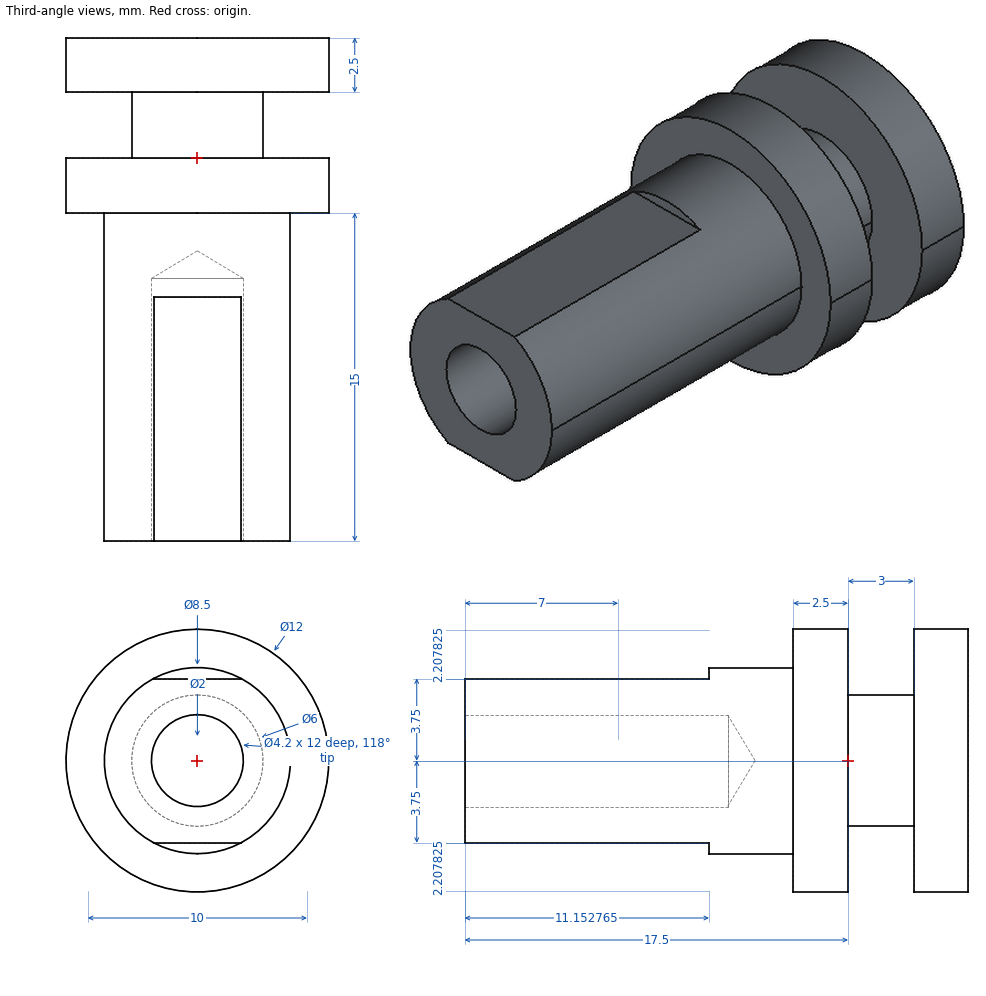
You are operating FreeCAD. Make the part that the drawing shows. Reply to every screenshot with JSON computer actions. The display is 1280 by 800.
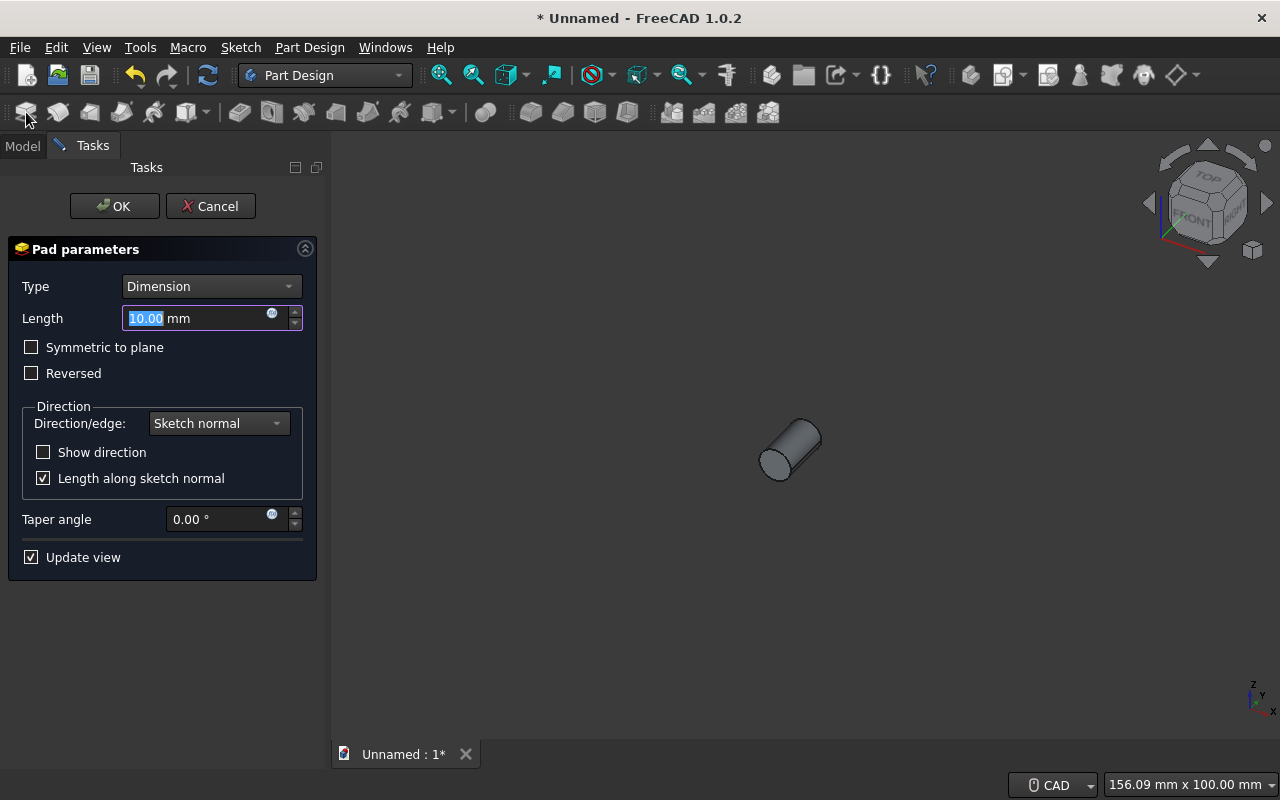
{"action": "type", "text": "3"}
{"action": "key", "text": "Tab"}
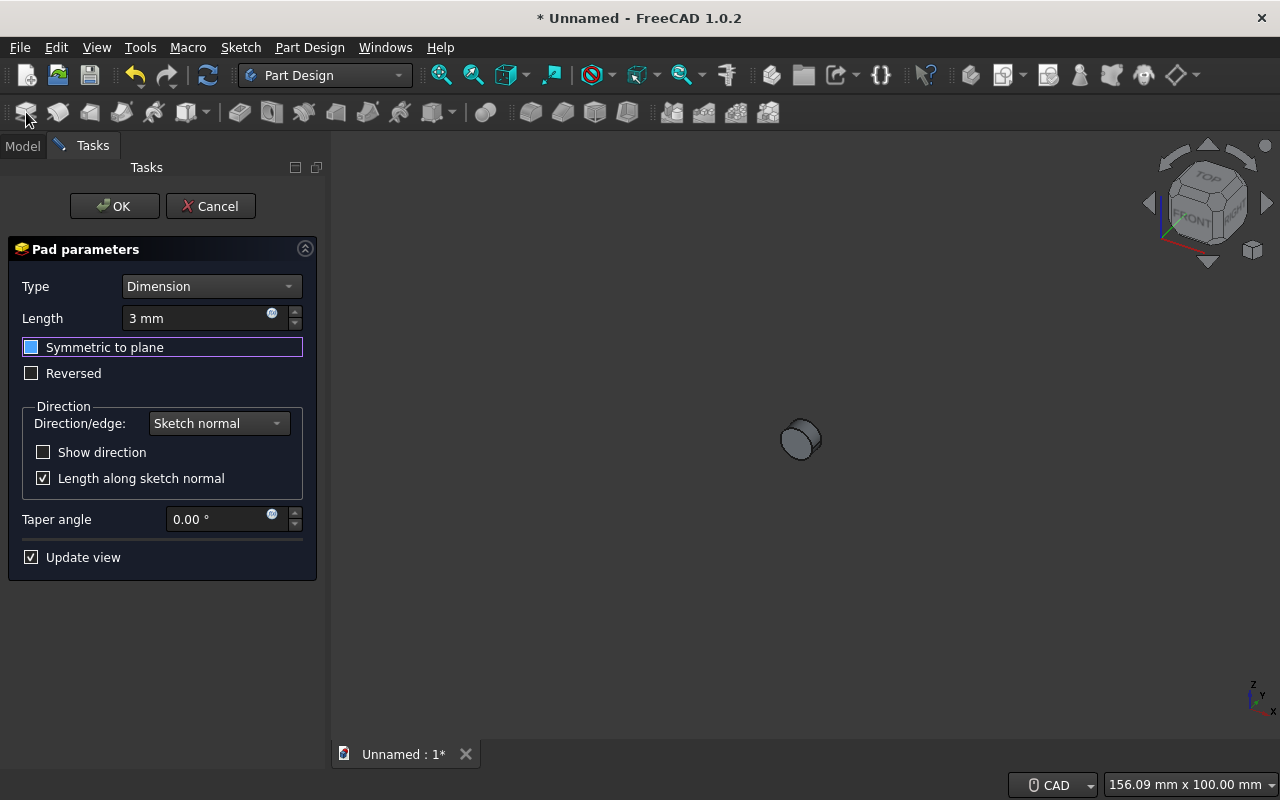
{"action": "left_click", "coordinate": [30, 373]}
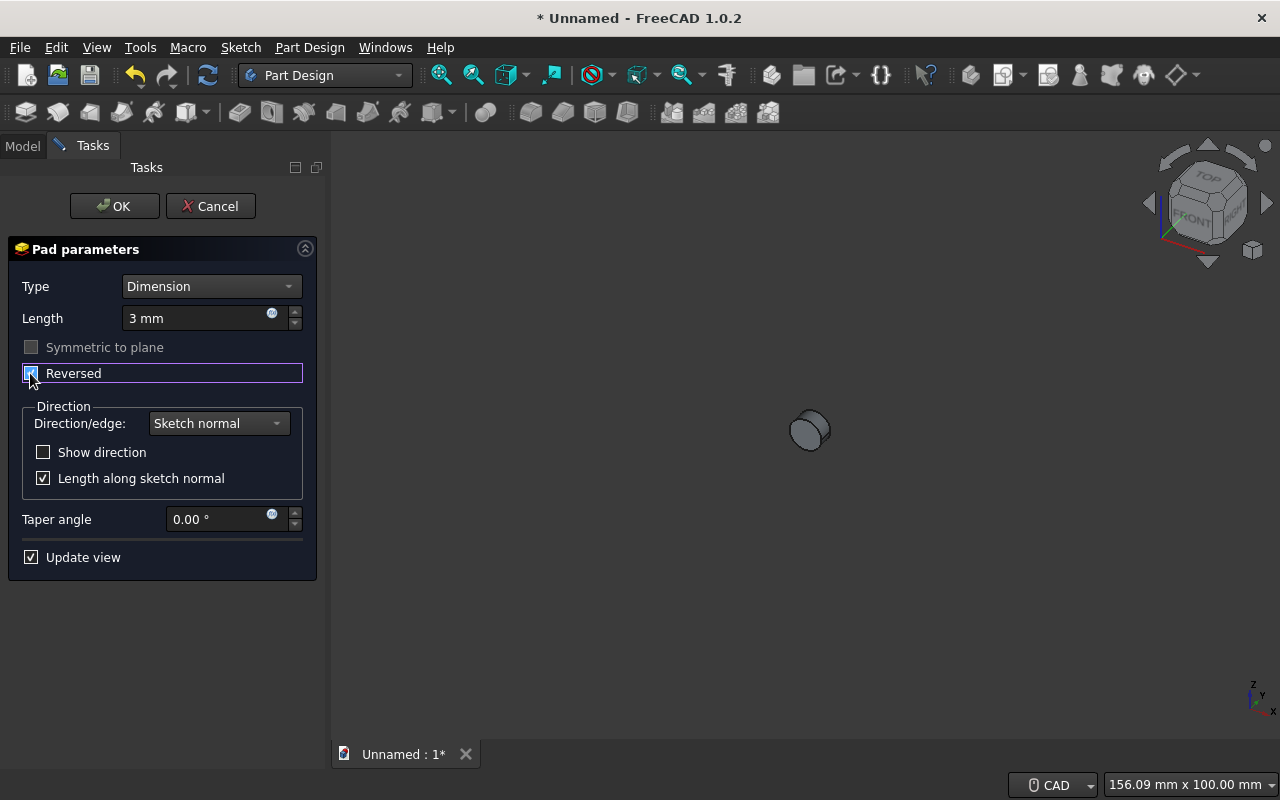
{"action": "left_click", "coordinate": [115, 206]}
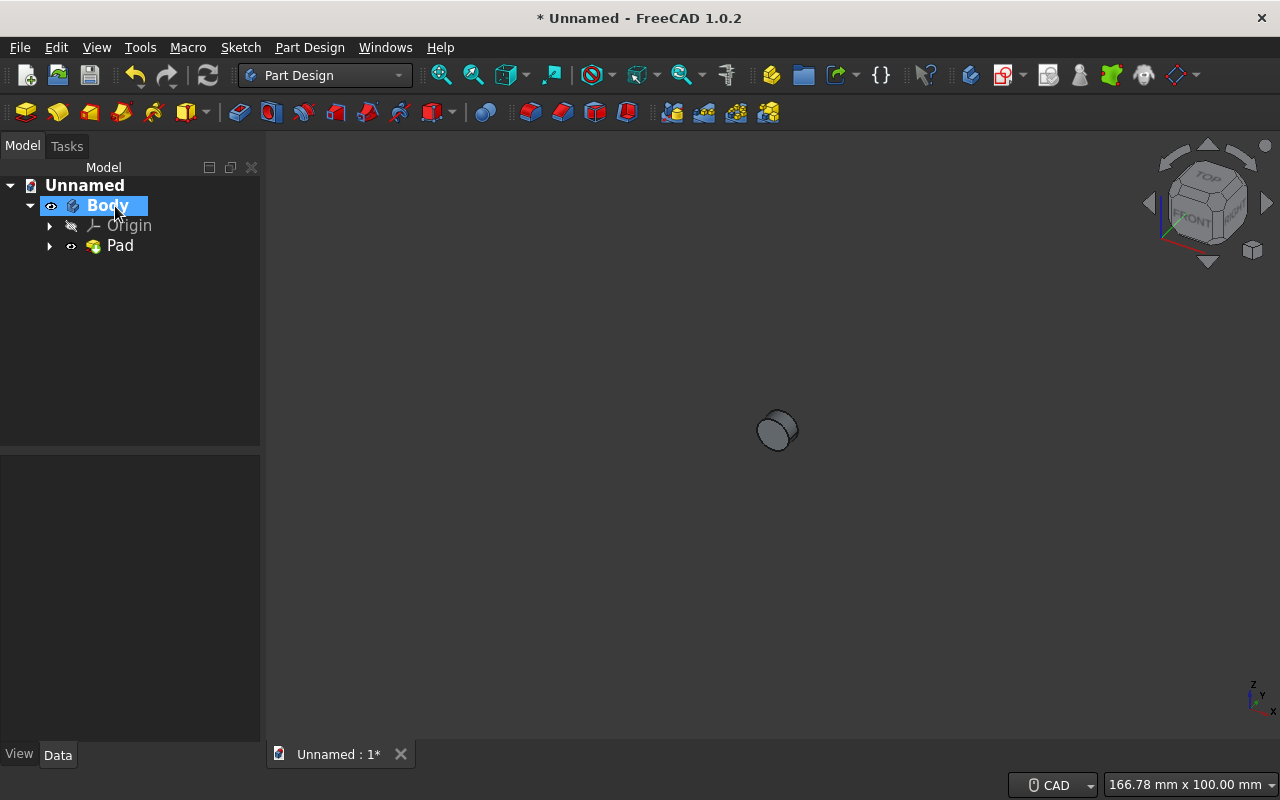
{"action": "key", "text": "v f"}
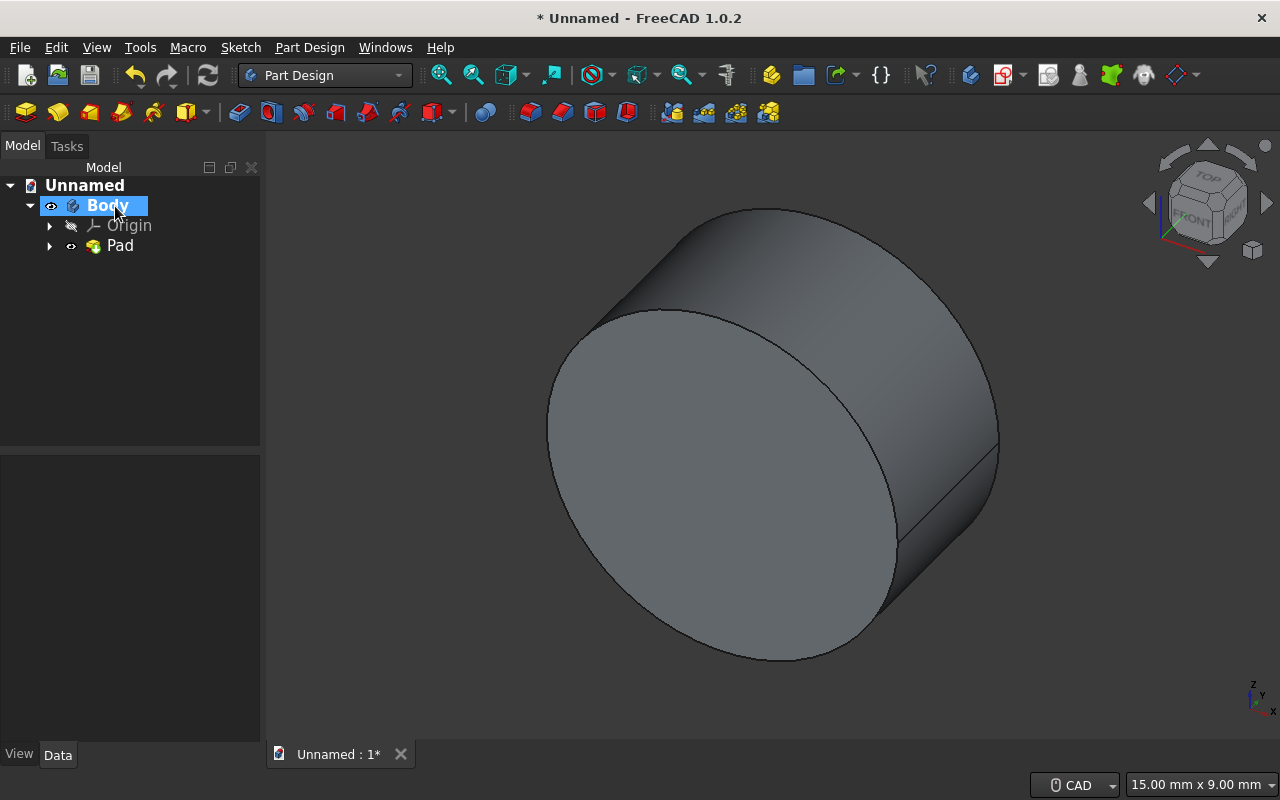
{"action": "key", "text": "4"}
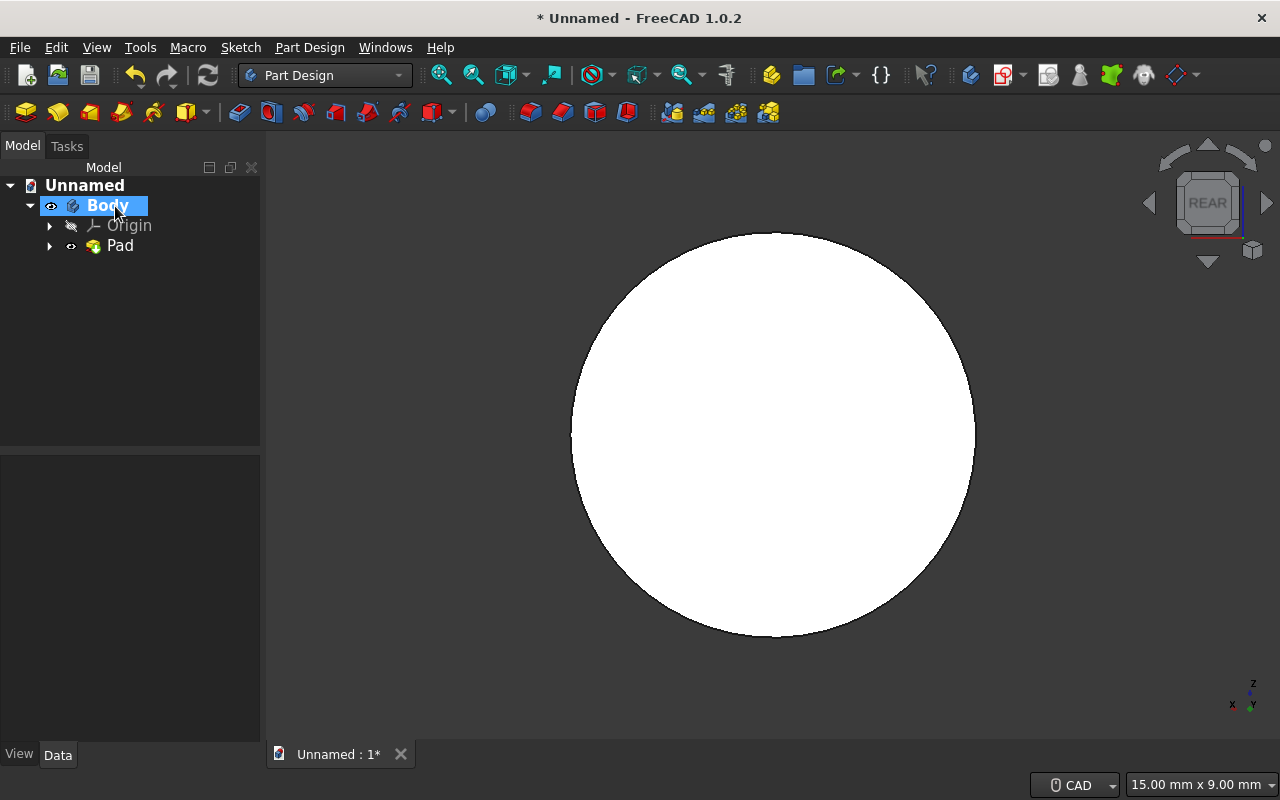
{"action": "left_click", "coordinate": [773, 434]}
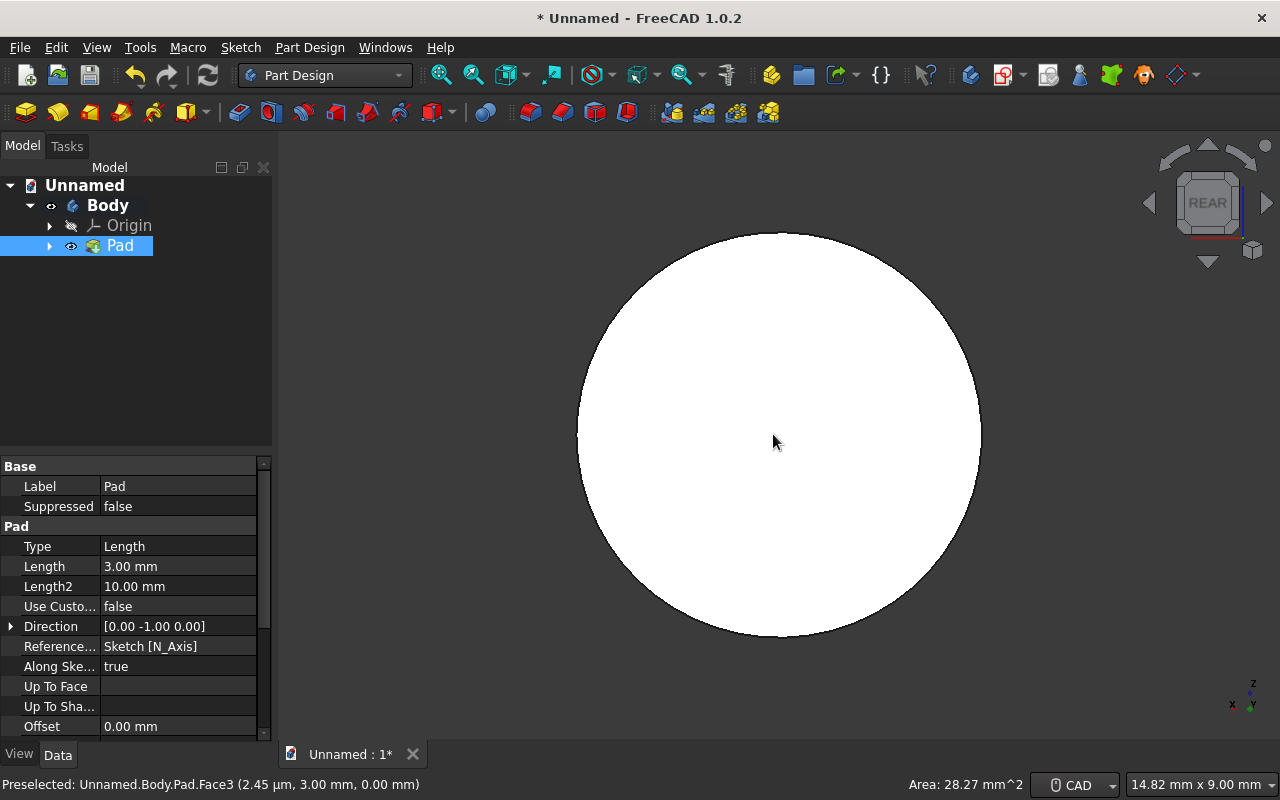
{"action": "left_click", "coordinate": [1004, 76]}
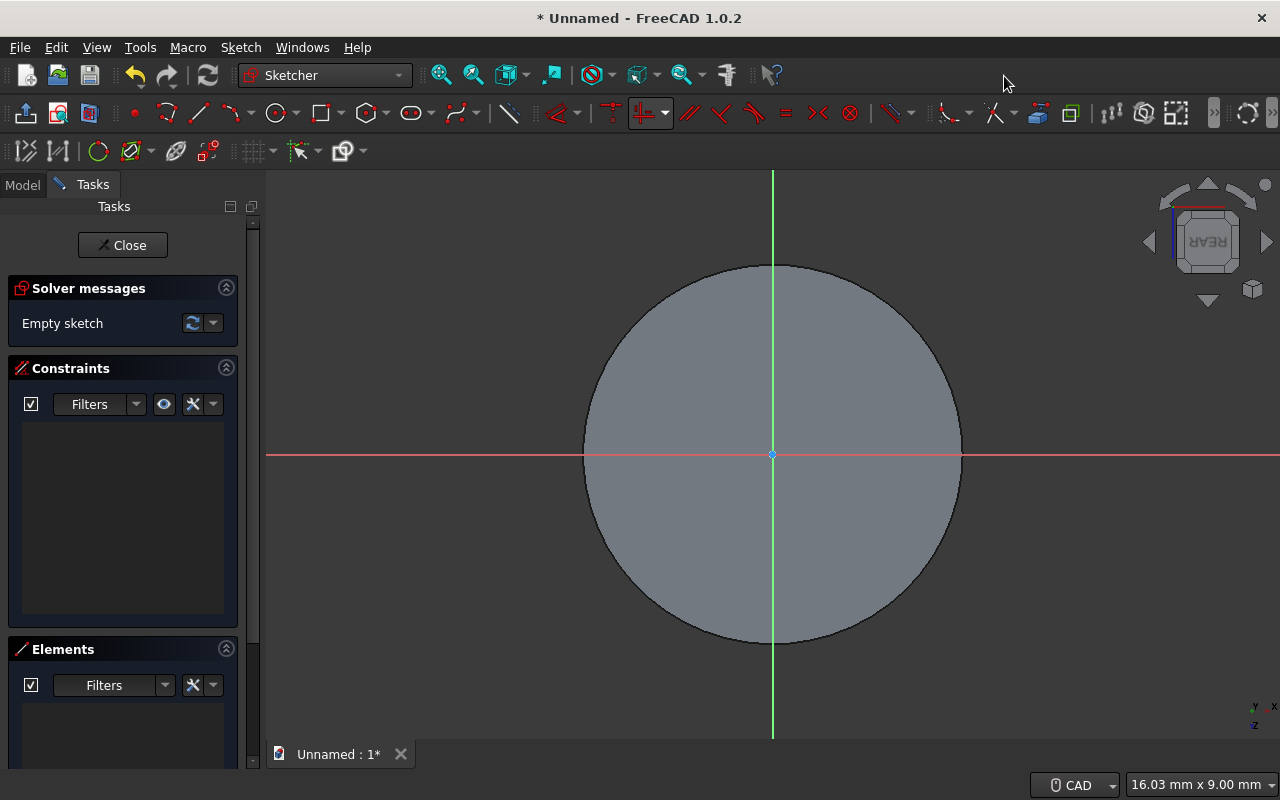
{"action": "scroll", "coordinate": [649, 454], "scroll_direction": "down", "scroll_amount": 4}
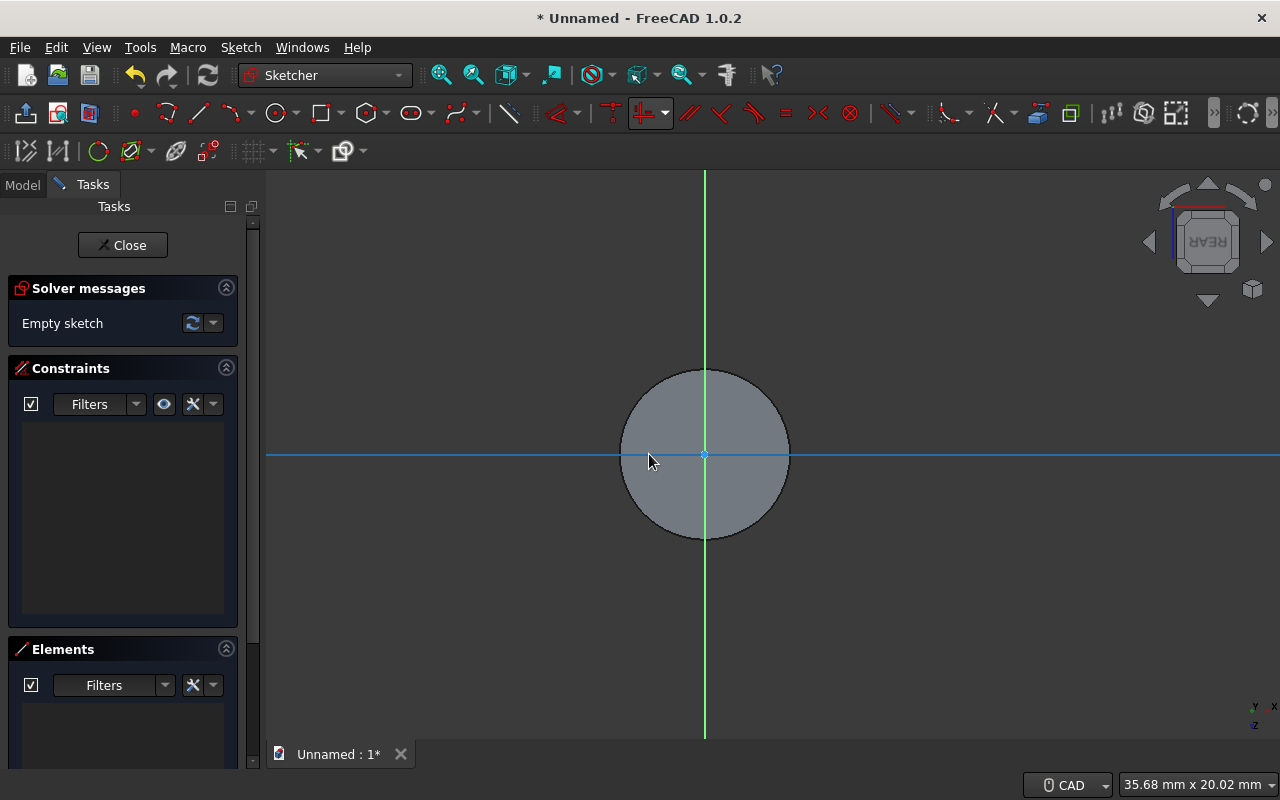
{"action": "key", "text": "g c"}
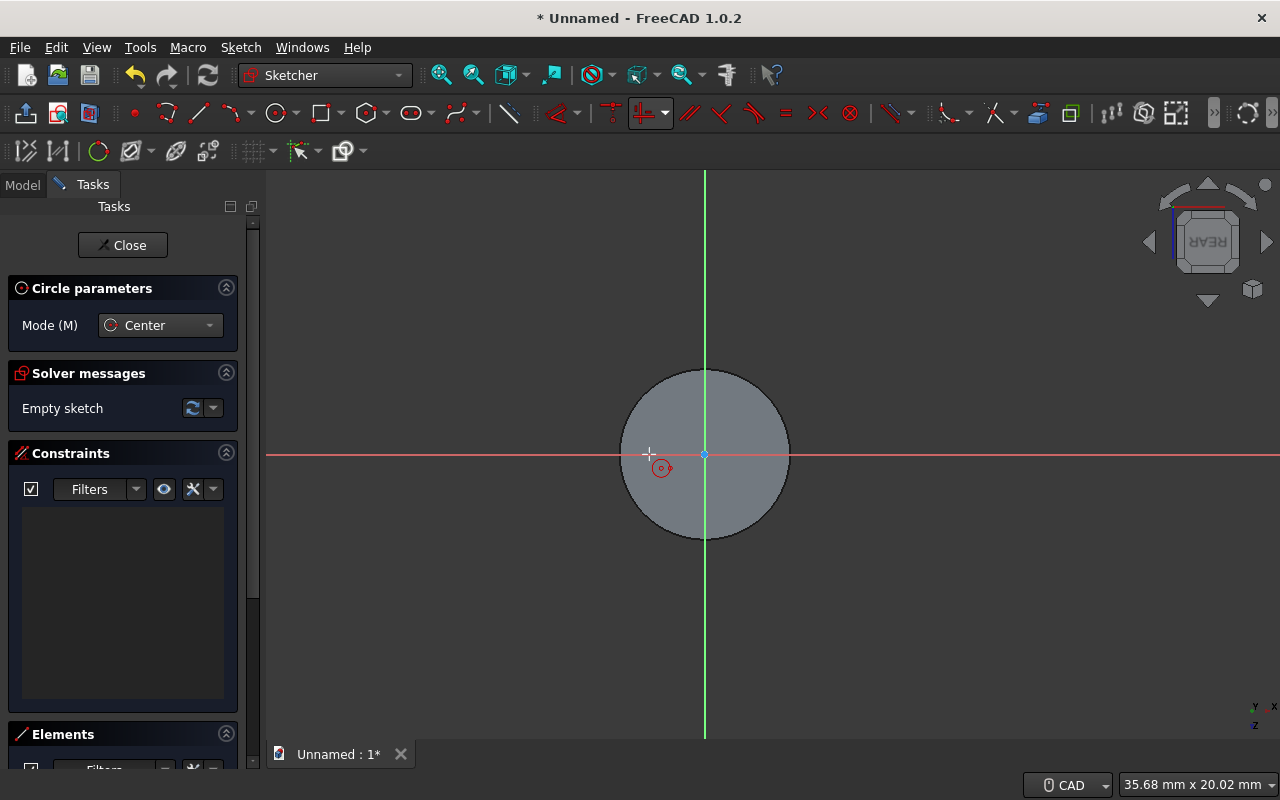
{"action": "left_click", "coordinate": [705, 455]}
{"action": "mouse_move", "coordinate": [825, 334]}